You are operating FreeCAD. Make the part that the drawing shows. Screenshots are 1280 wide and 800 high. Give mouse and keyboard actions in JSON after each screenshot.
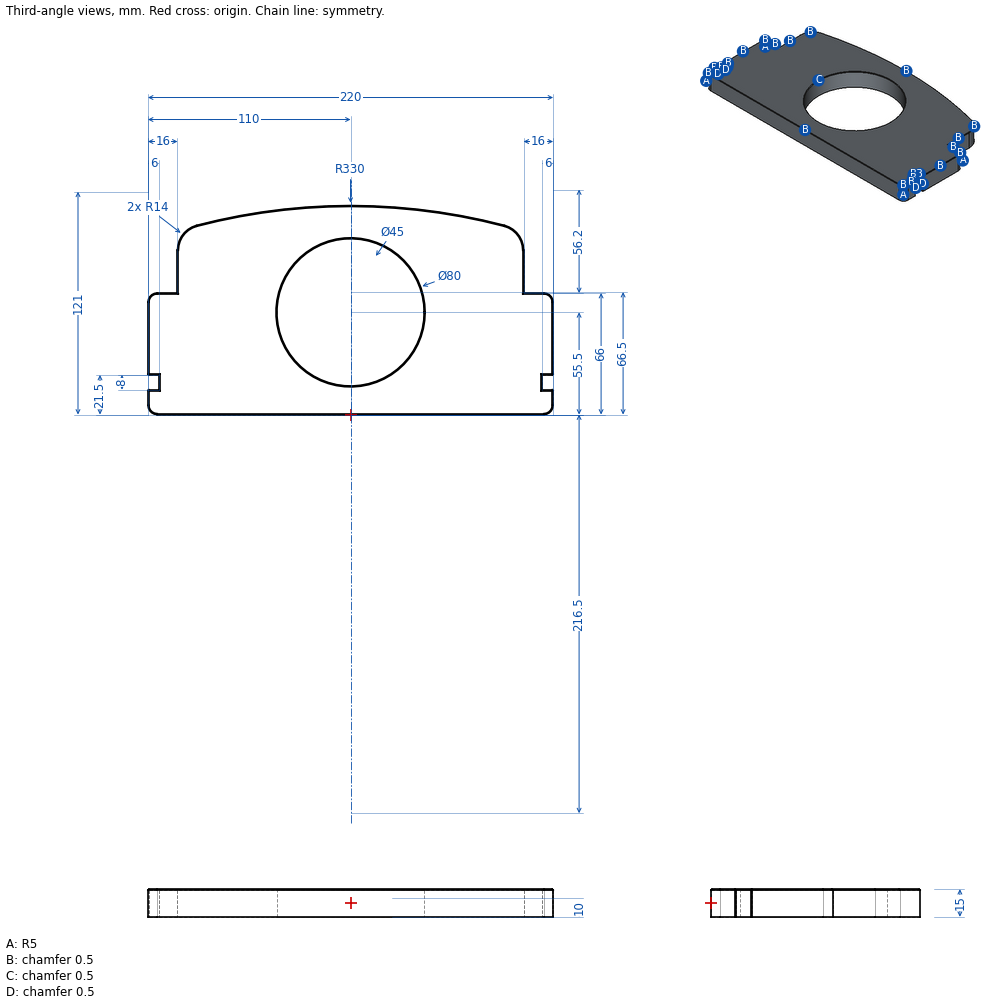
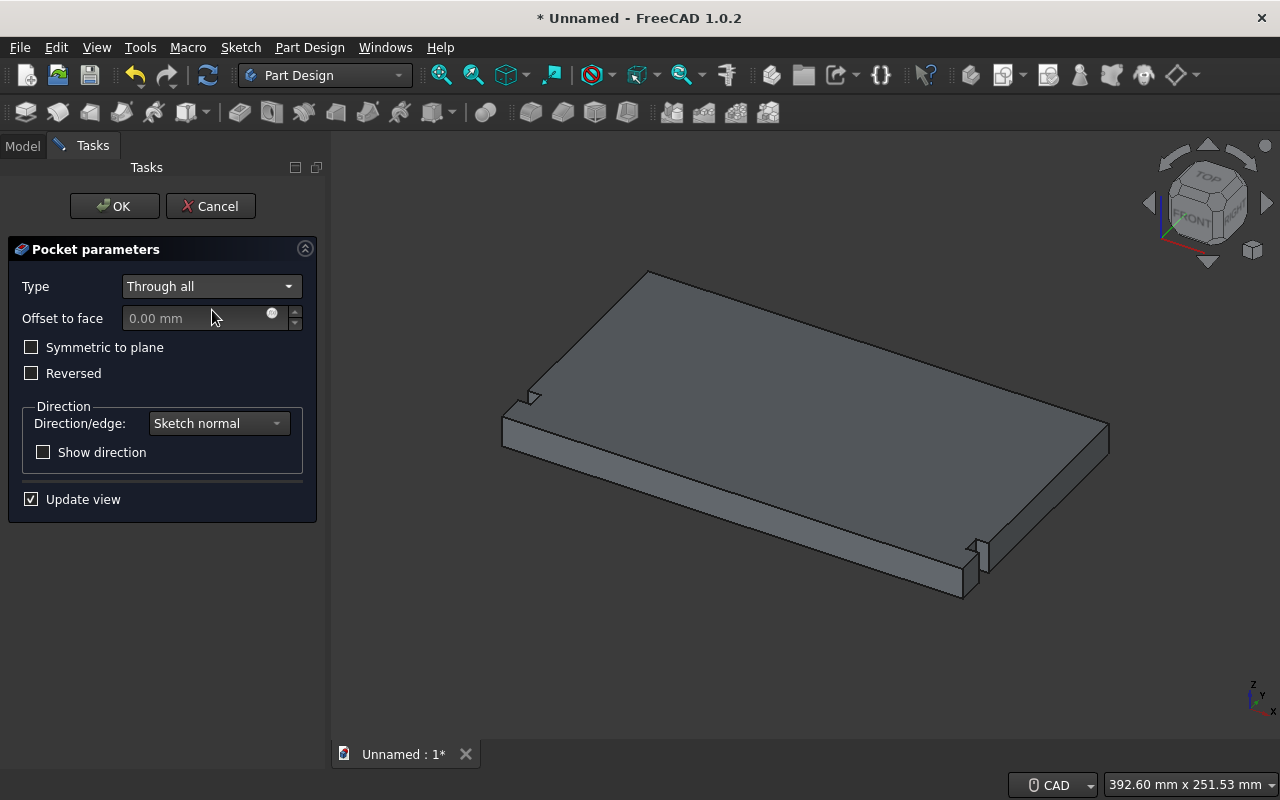
{"action": "left_click", "coordinate": [115, 206]}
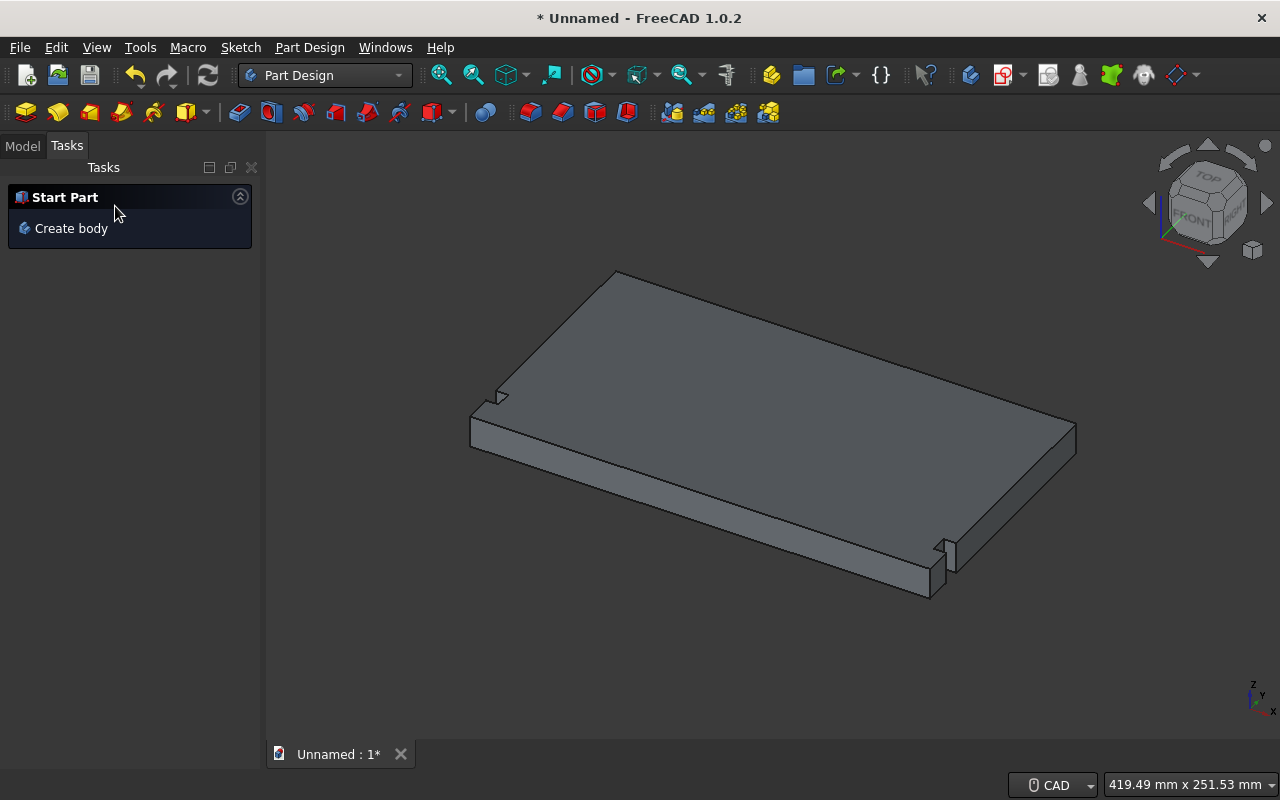
{"action": "key", "text": "5"}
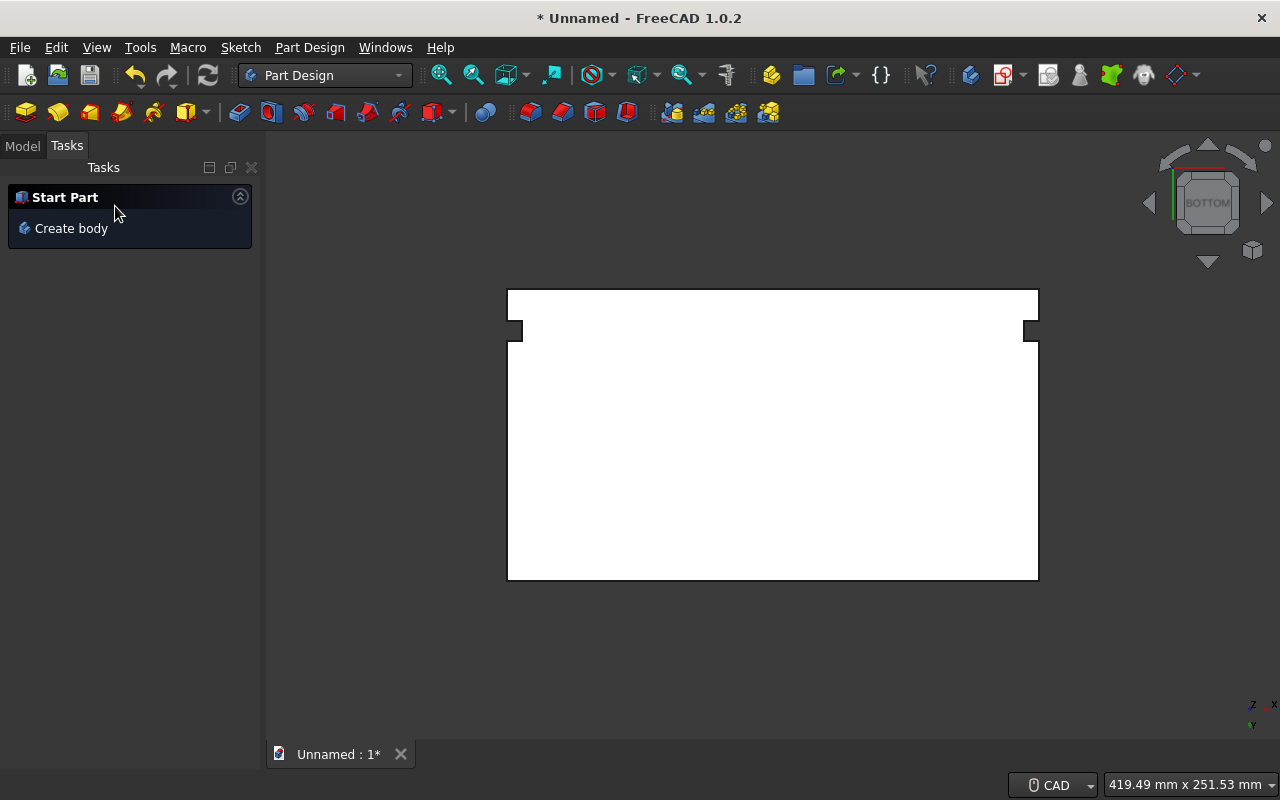
{"action": "left_click", "coordinate": [849, 434]}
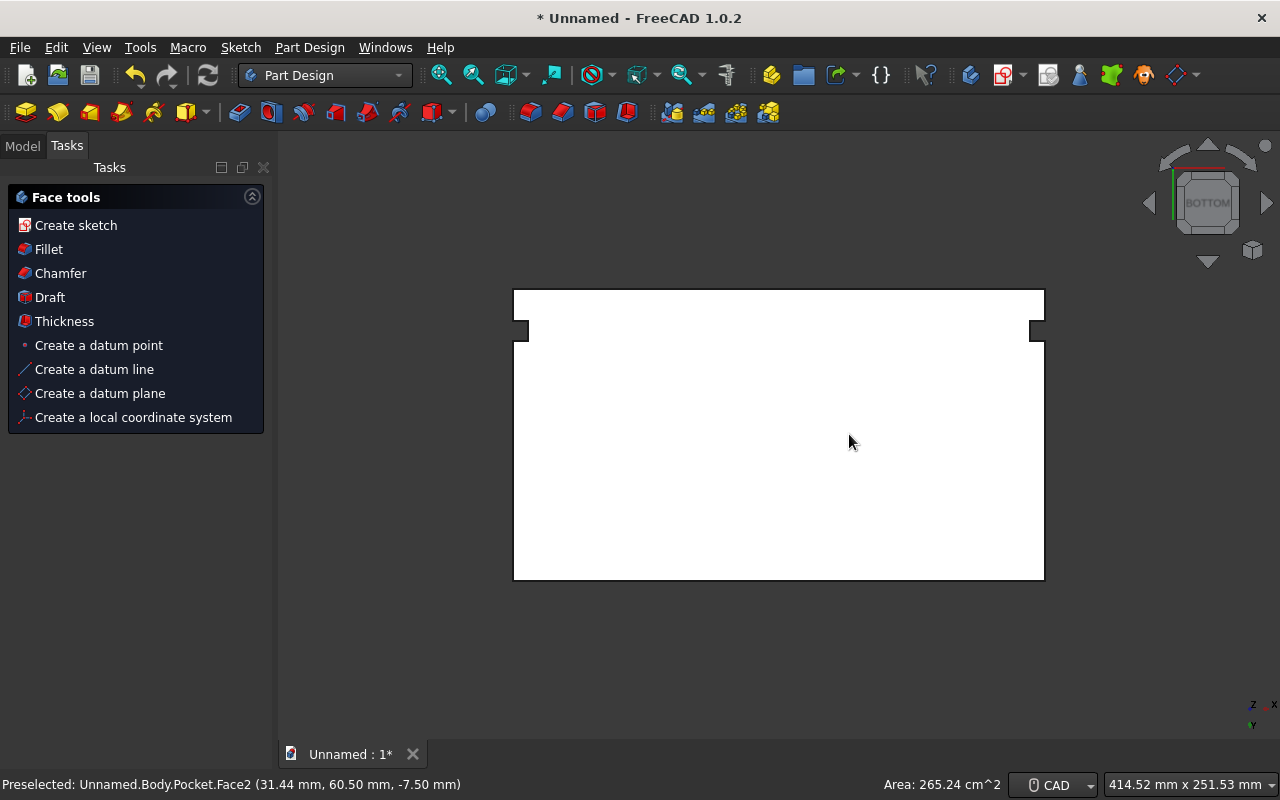
{"action": "left_click", "coordinate": [1004, 76]}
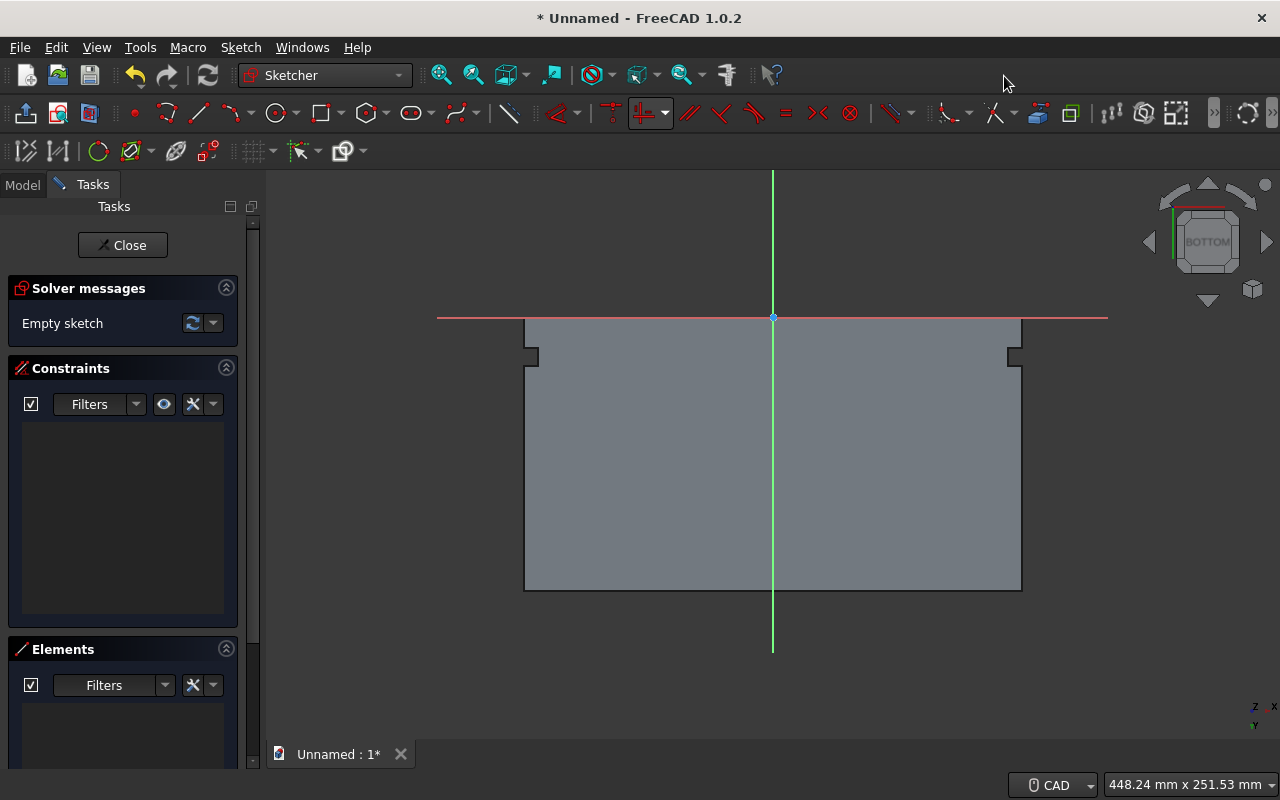
{"action": "scroll", "coordinate": [856, 374], "scroll_direction": "up", "scroll_amount": 3}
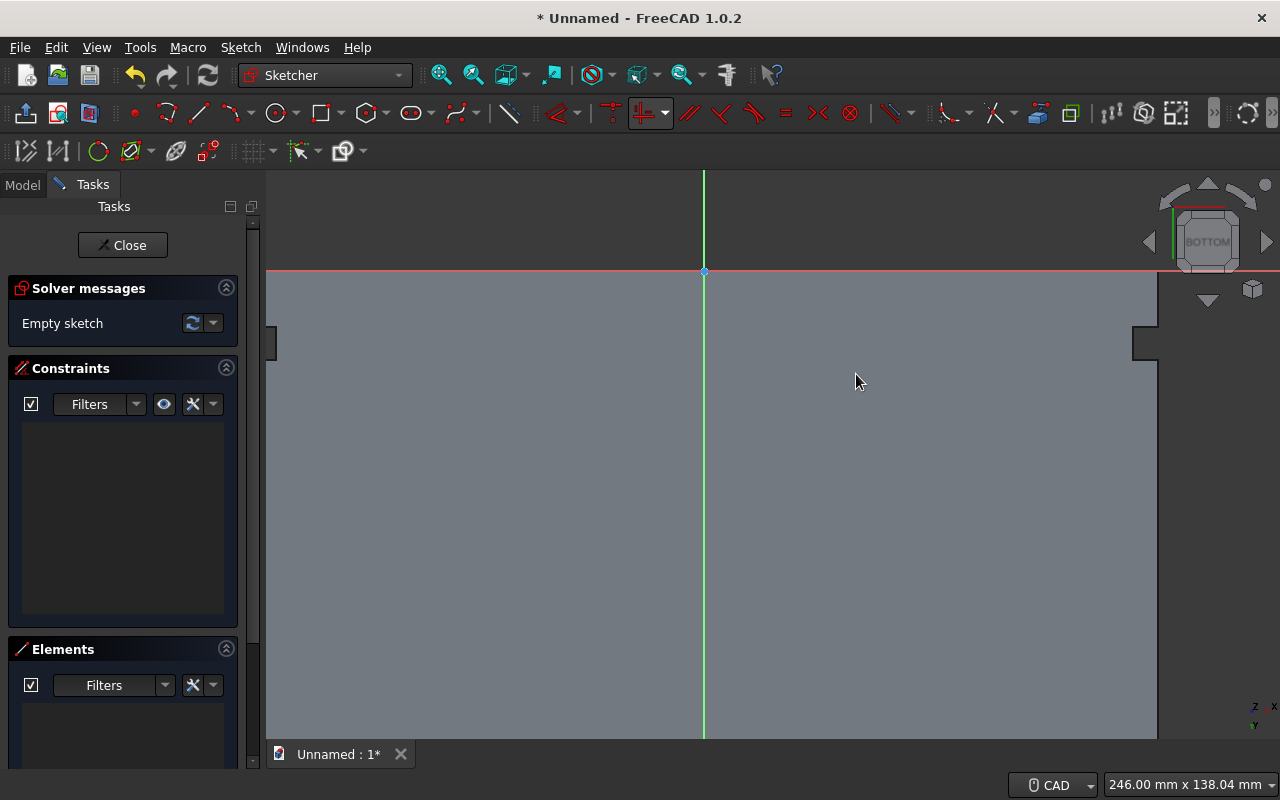
{"action": "left_click", "coordinate": [276, 114]}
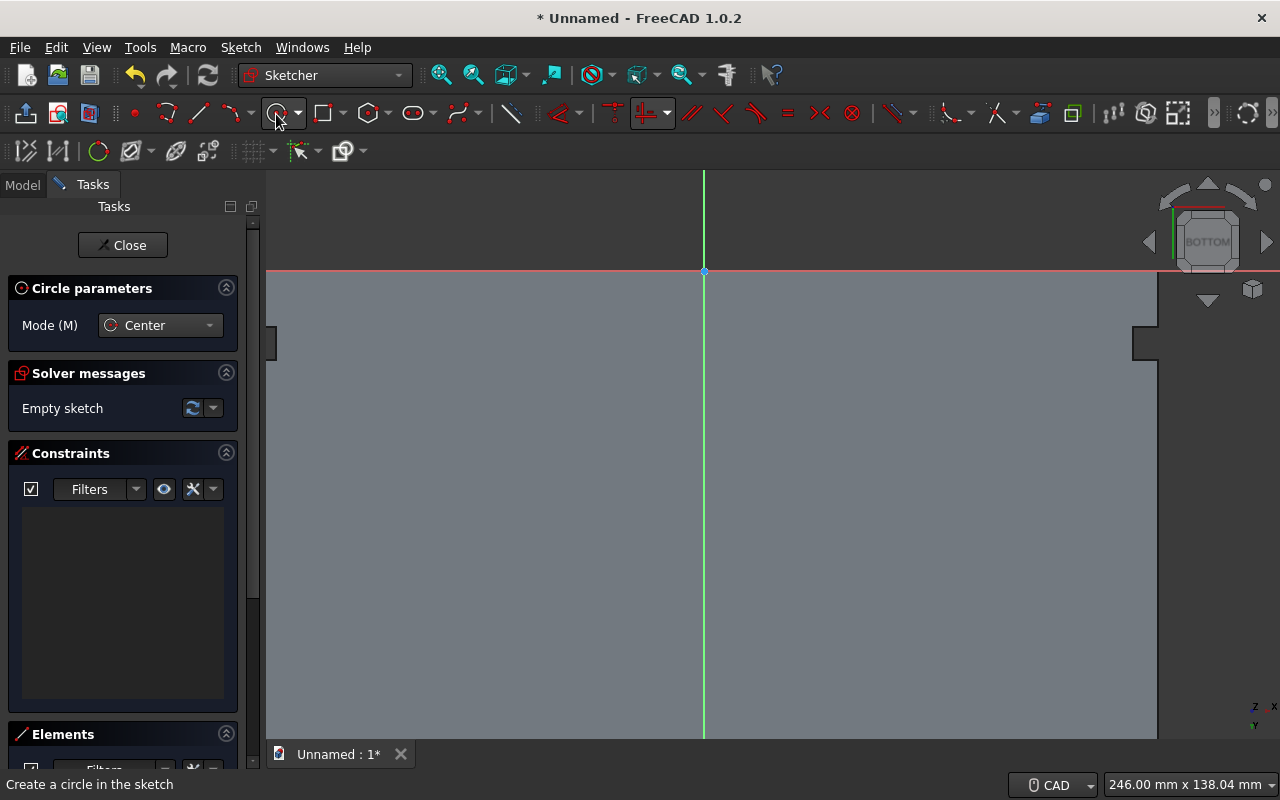
{"action": "left_click", "coordinate": [704, 545]}
{"action": "mouse_move", "coordinate": [770, 480]}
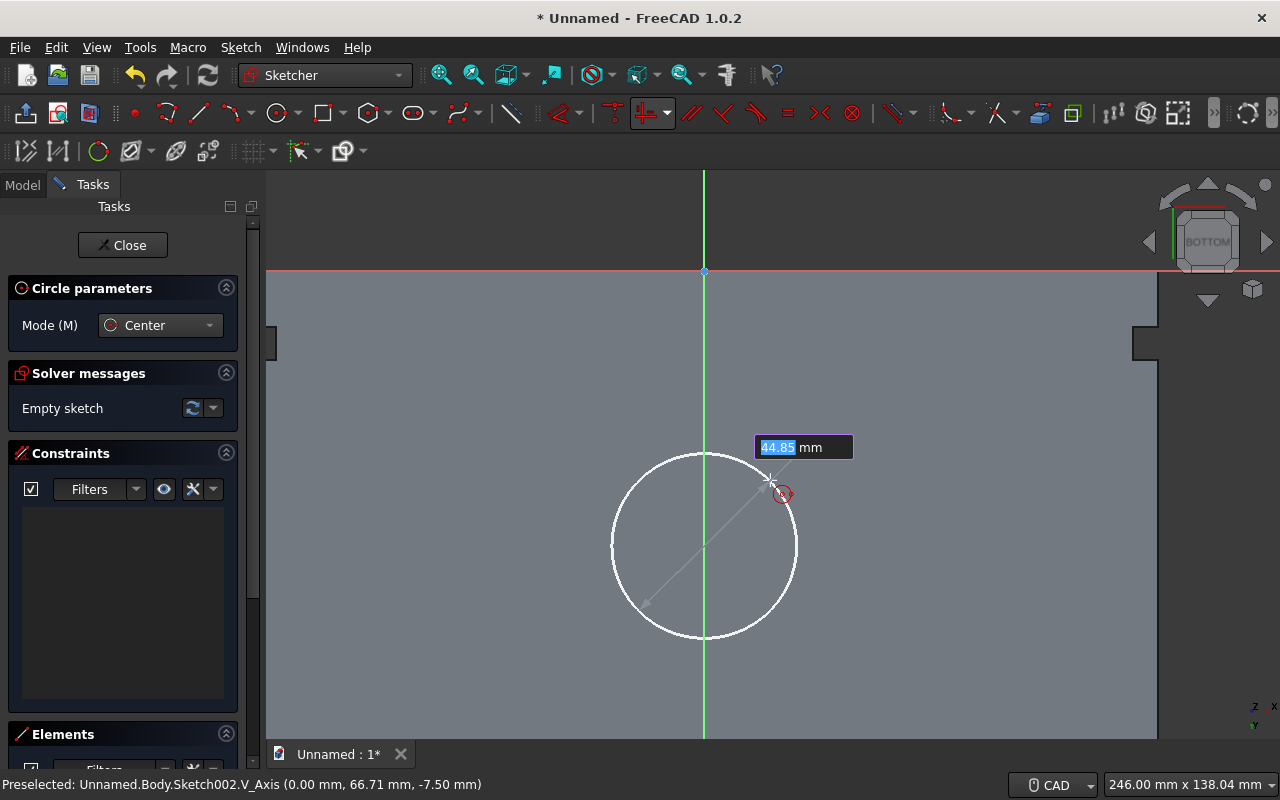
{"action": "type", "text": "45"}
{"action": "key", "text": "Return"}
{"action": "key", "text": "Escape"}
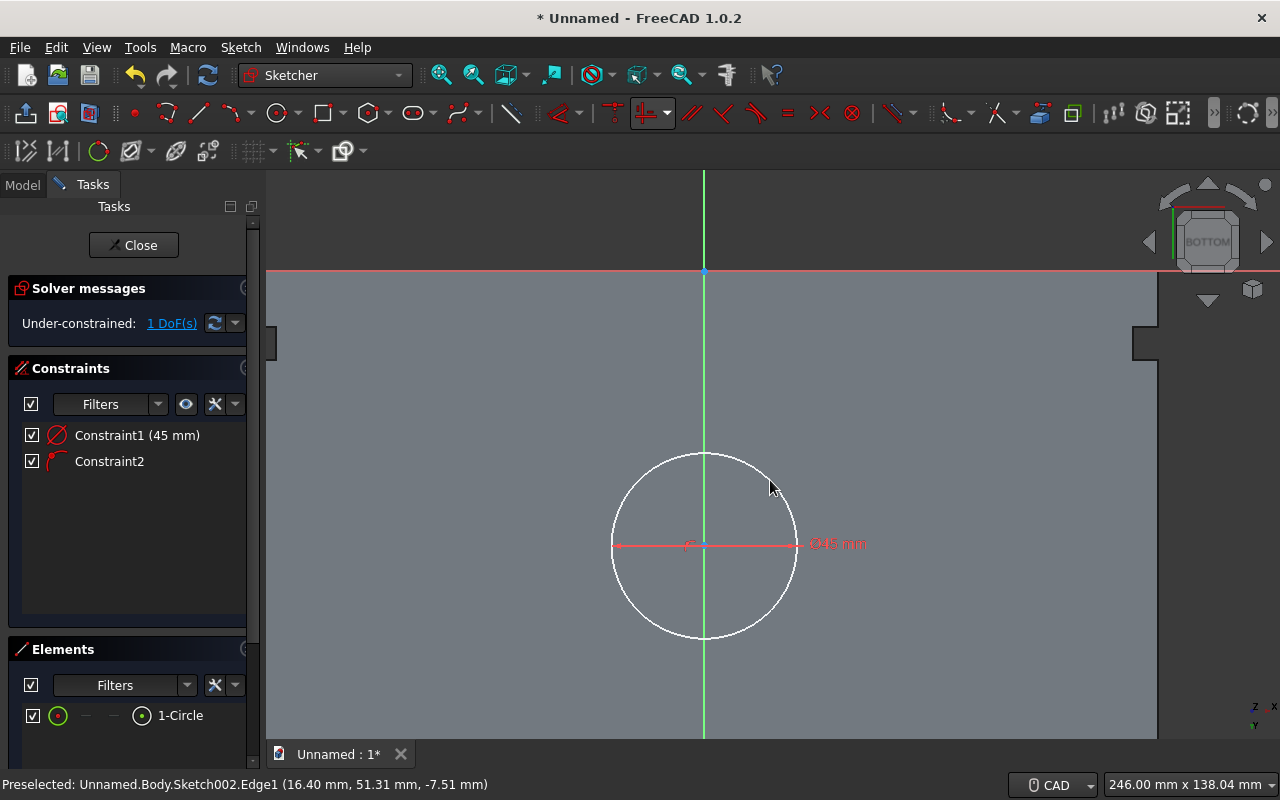
{"action": "left_click", "coordinate": [558, 114]}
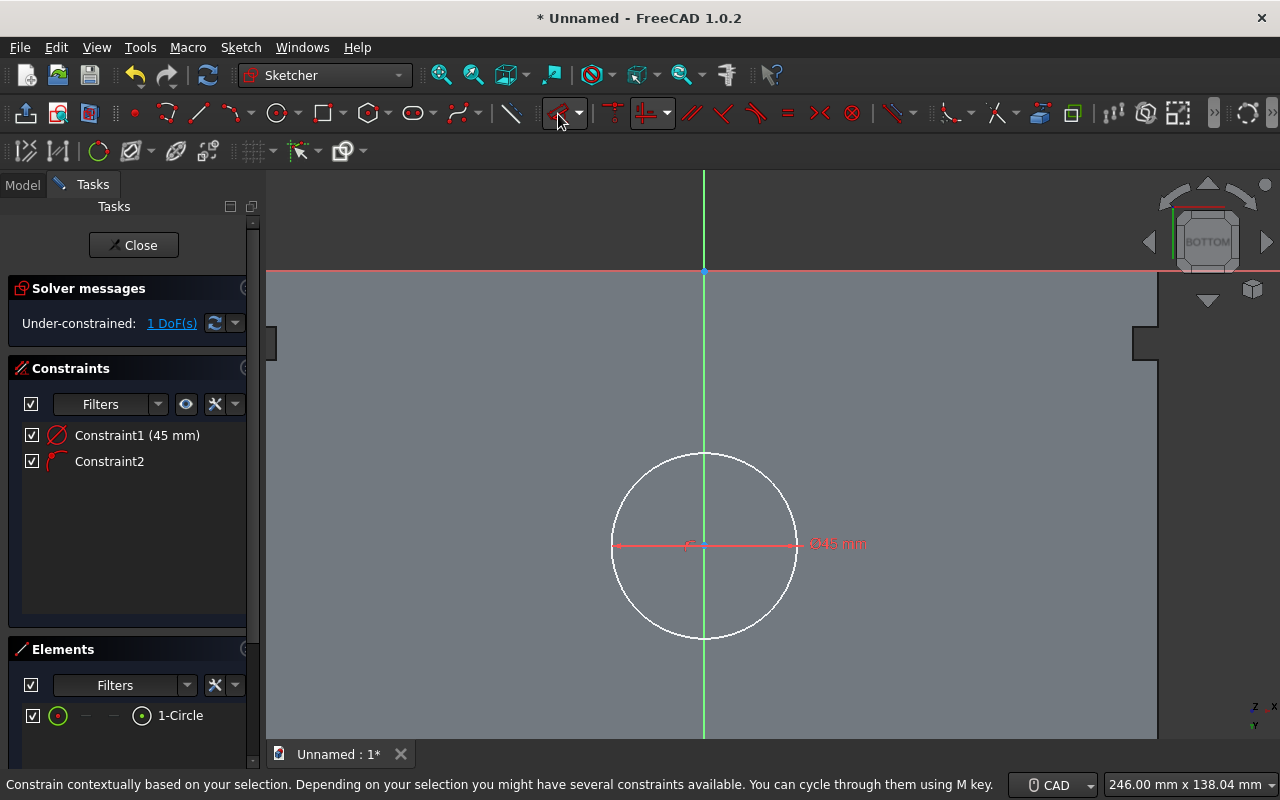
{"action": "left_click", "coordinate": [704, 546]}
{"action": "left_click", "coordinate": [738, 409]}